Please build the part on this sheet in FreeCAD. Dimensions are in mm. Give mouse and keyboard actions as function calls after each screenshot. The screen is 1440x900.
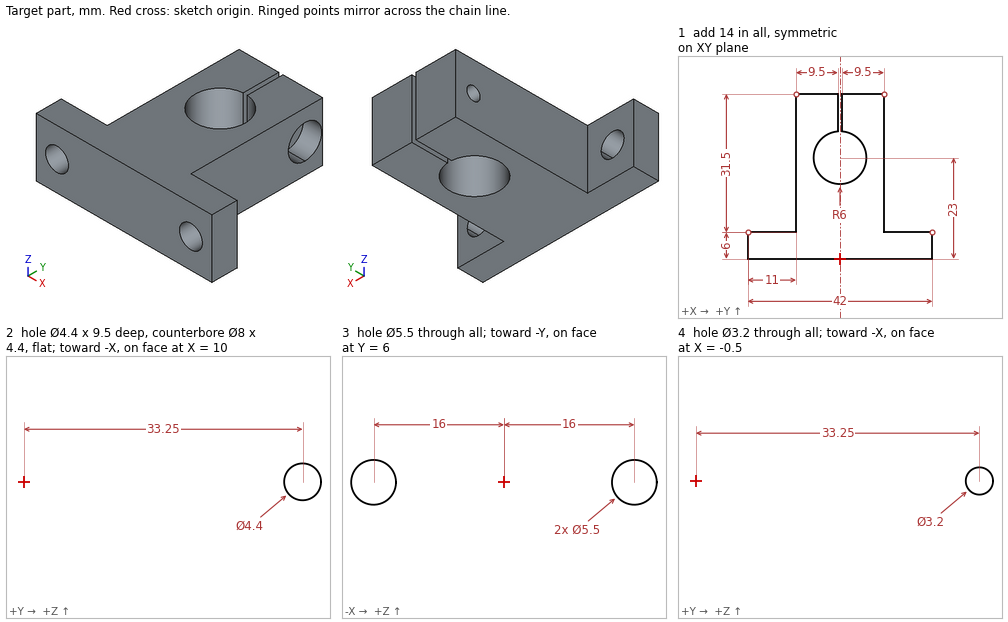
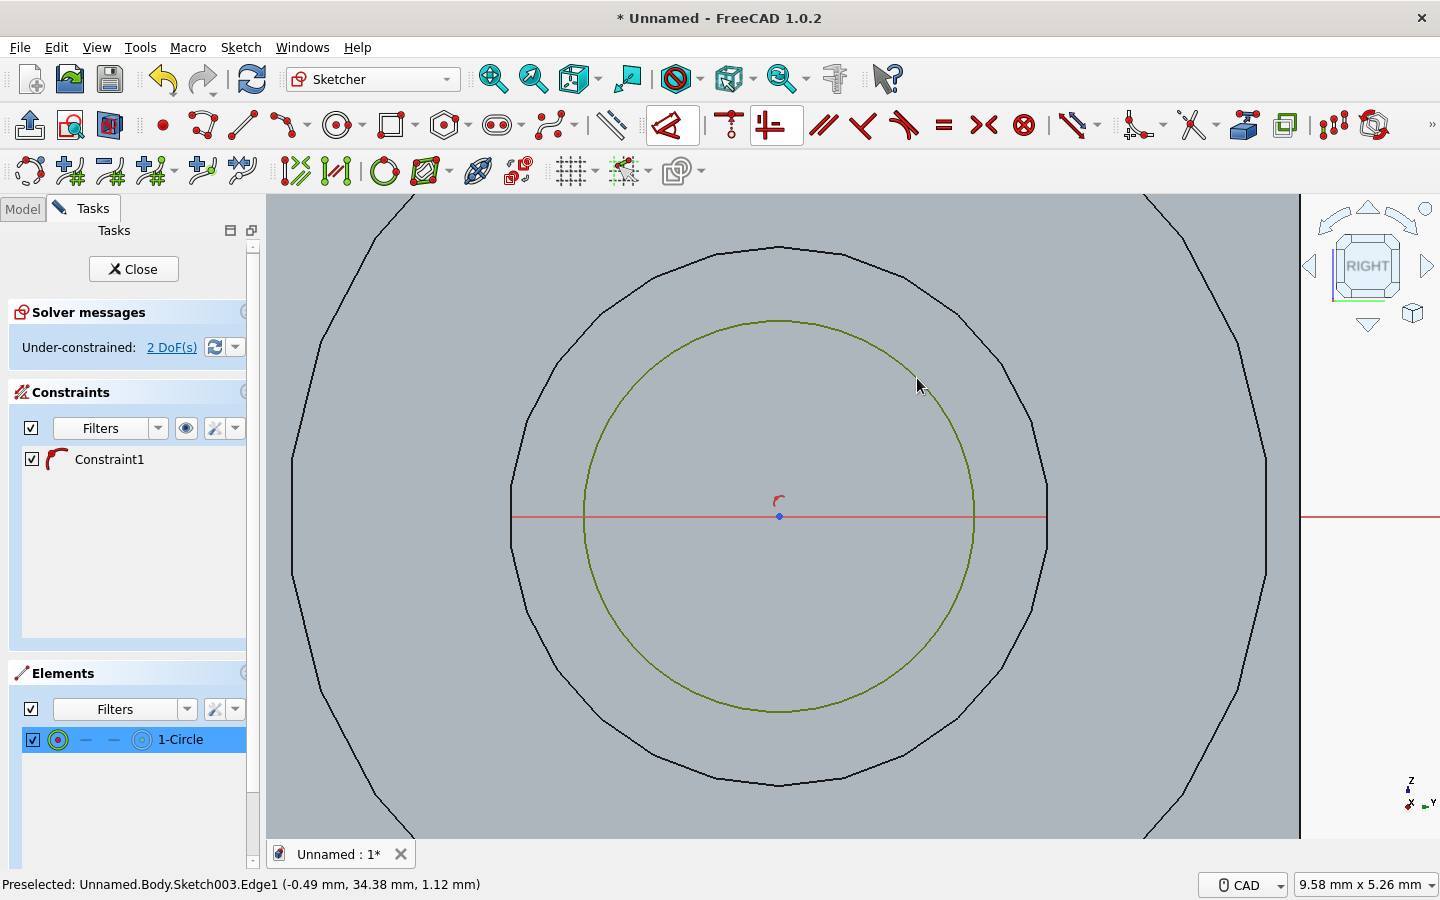
click(694, 126)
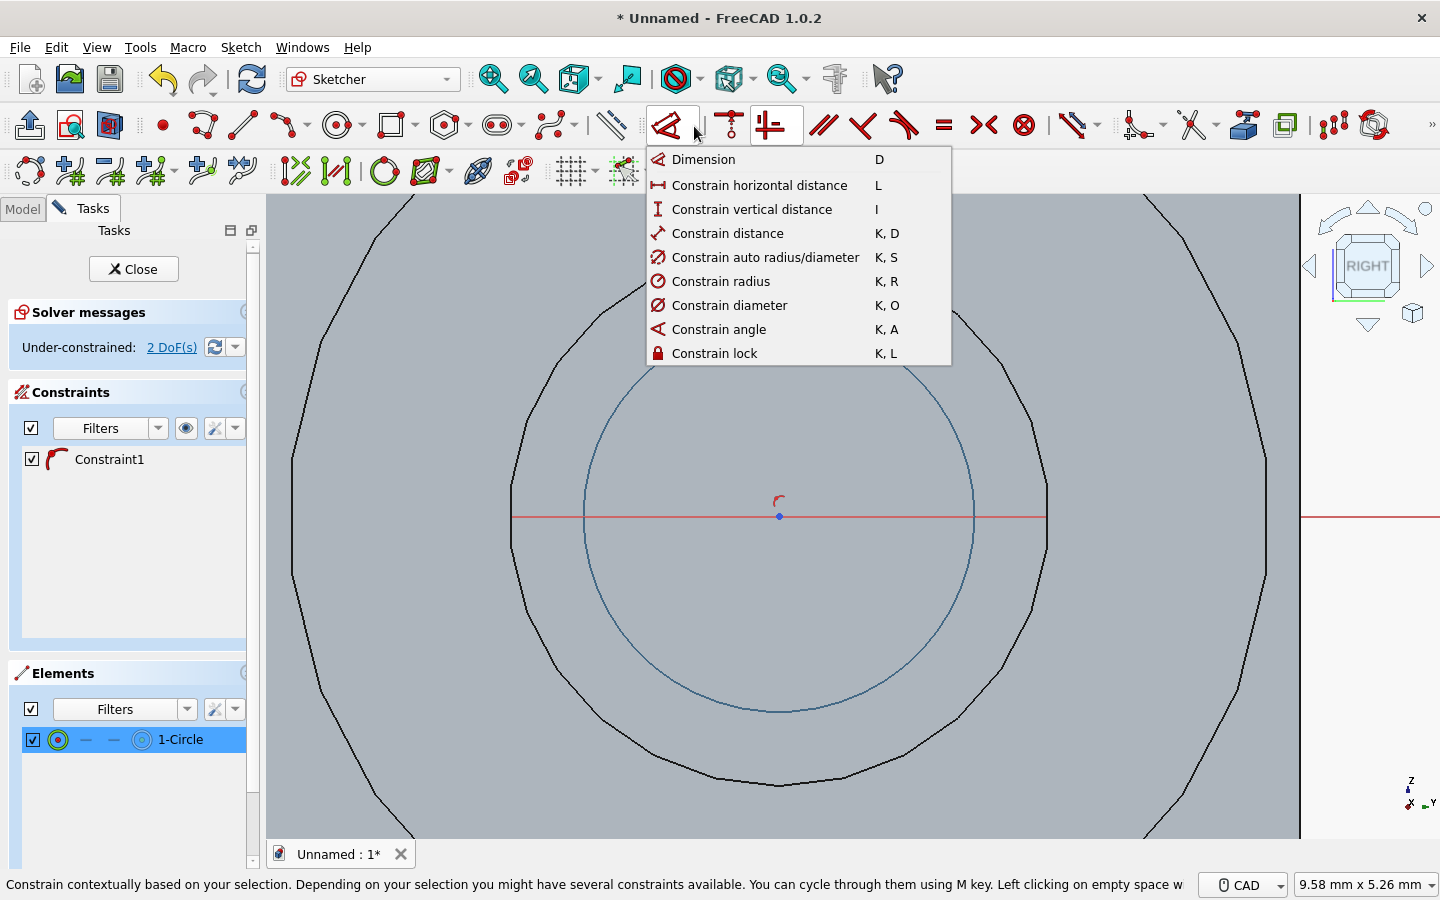
click(799, 305)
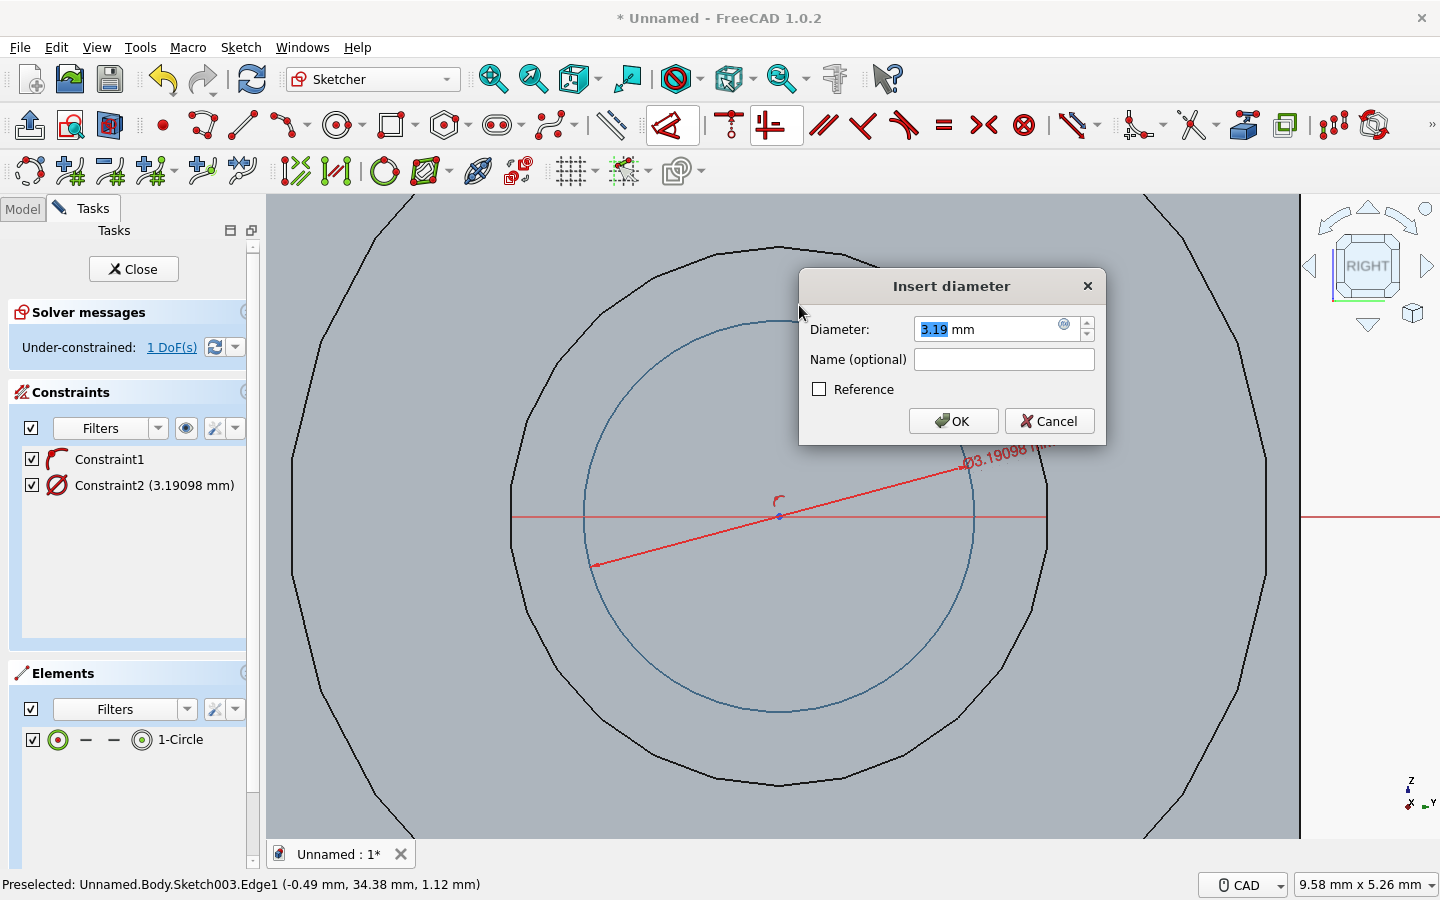
text(3.2)
key(Return)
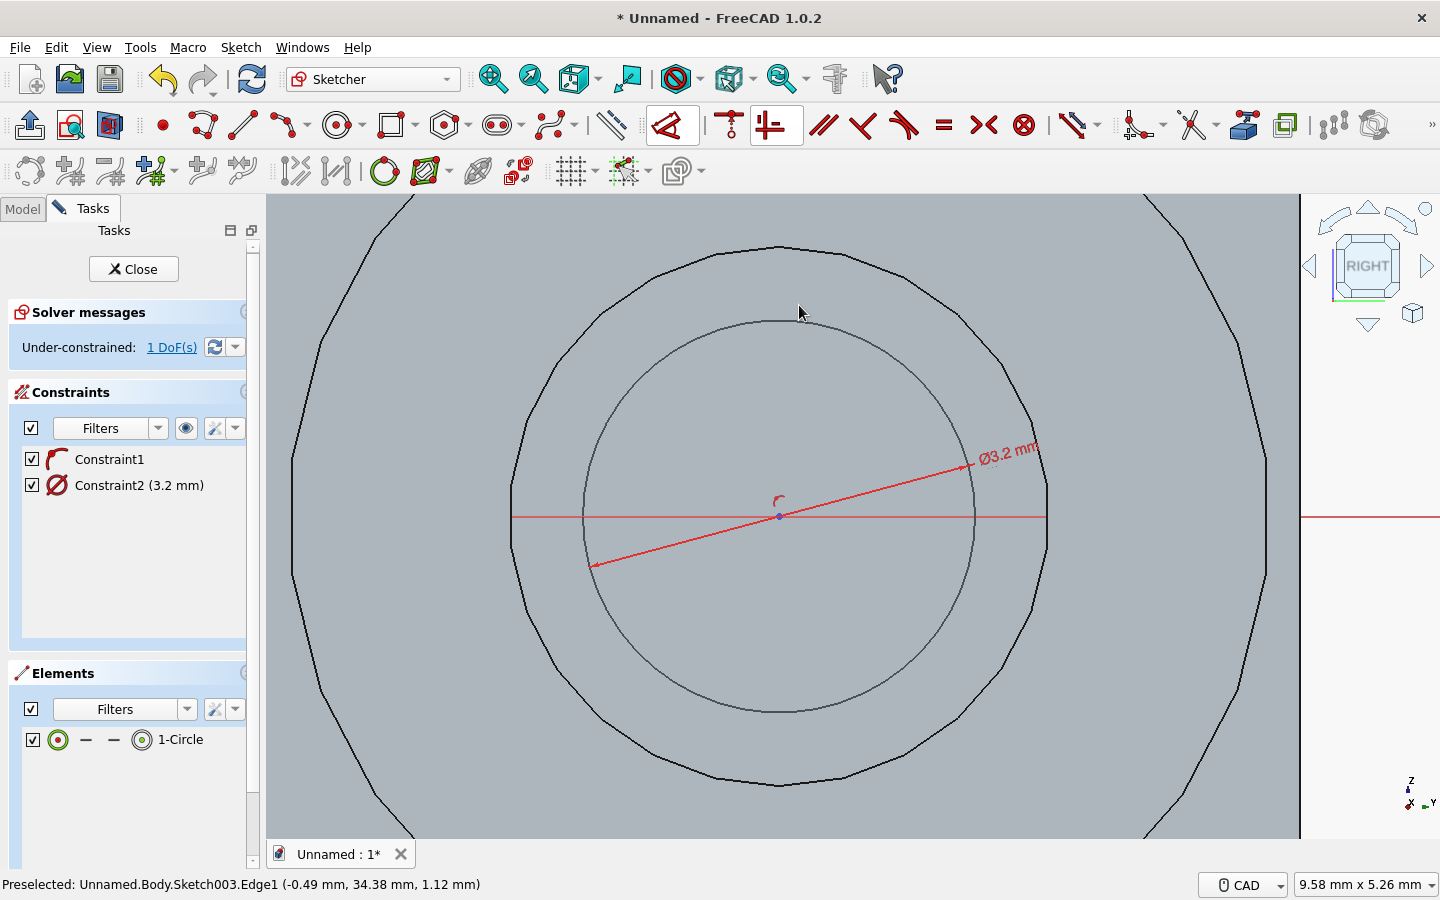
click(779, 516)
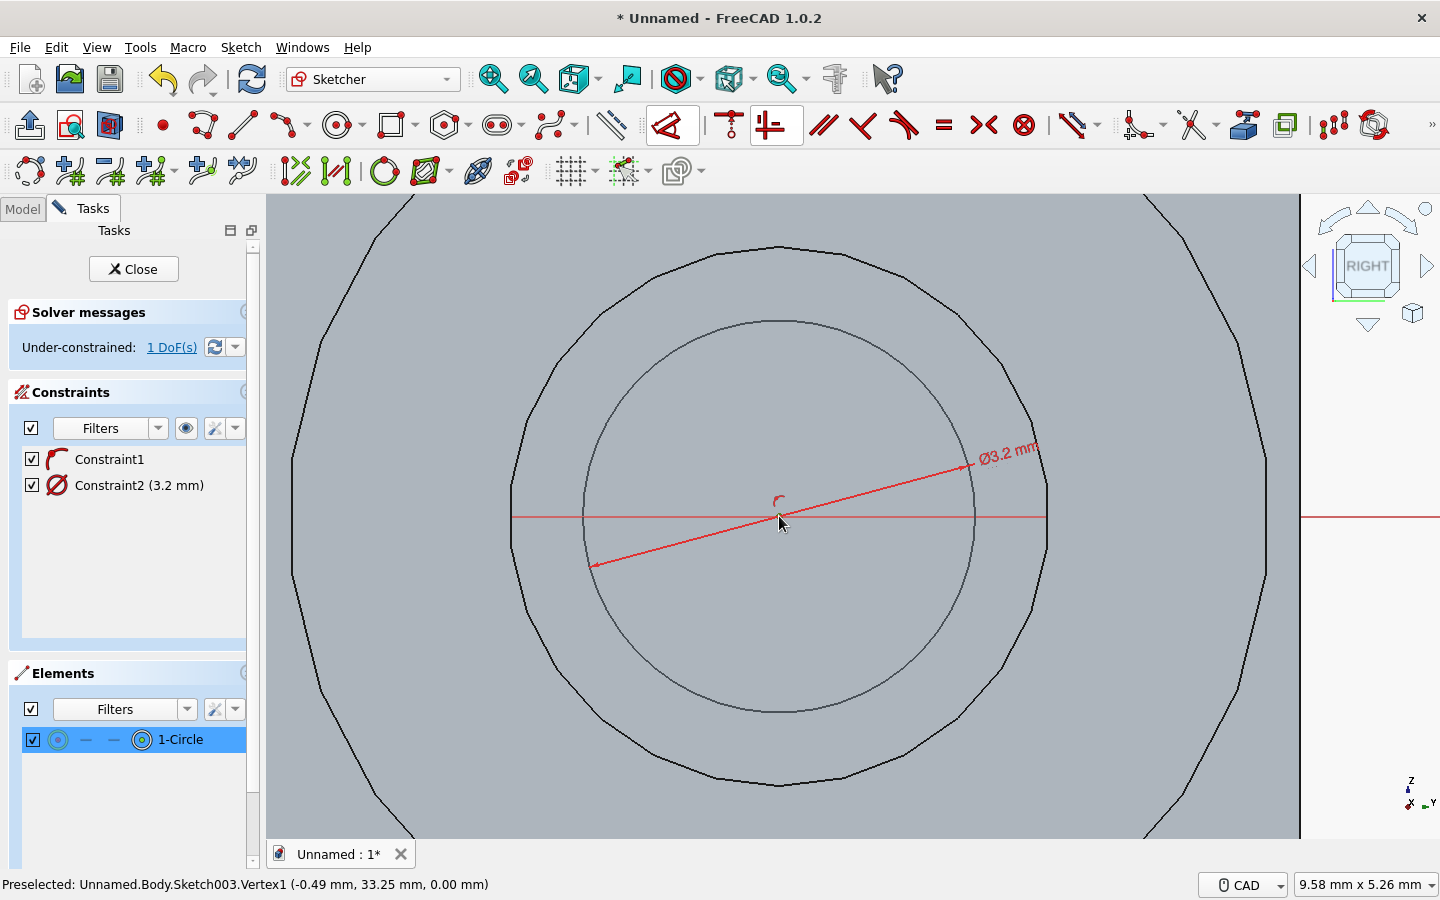
click(694, 126)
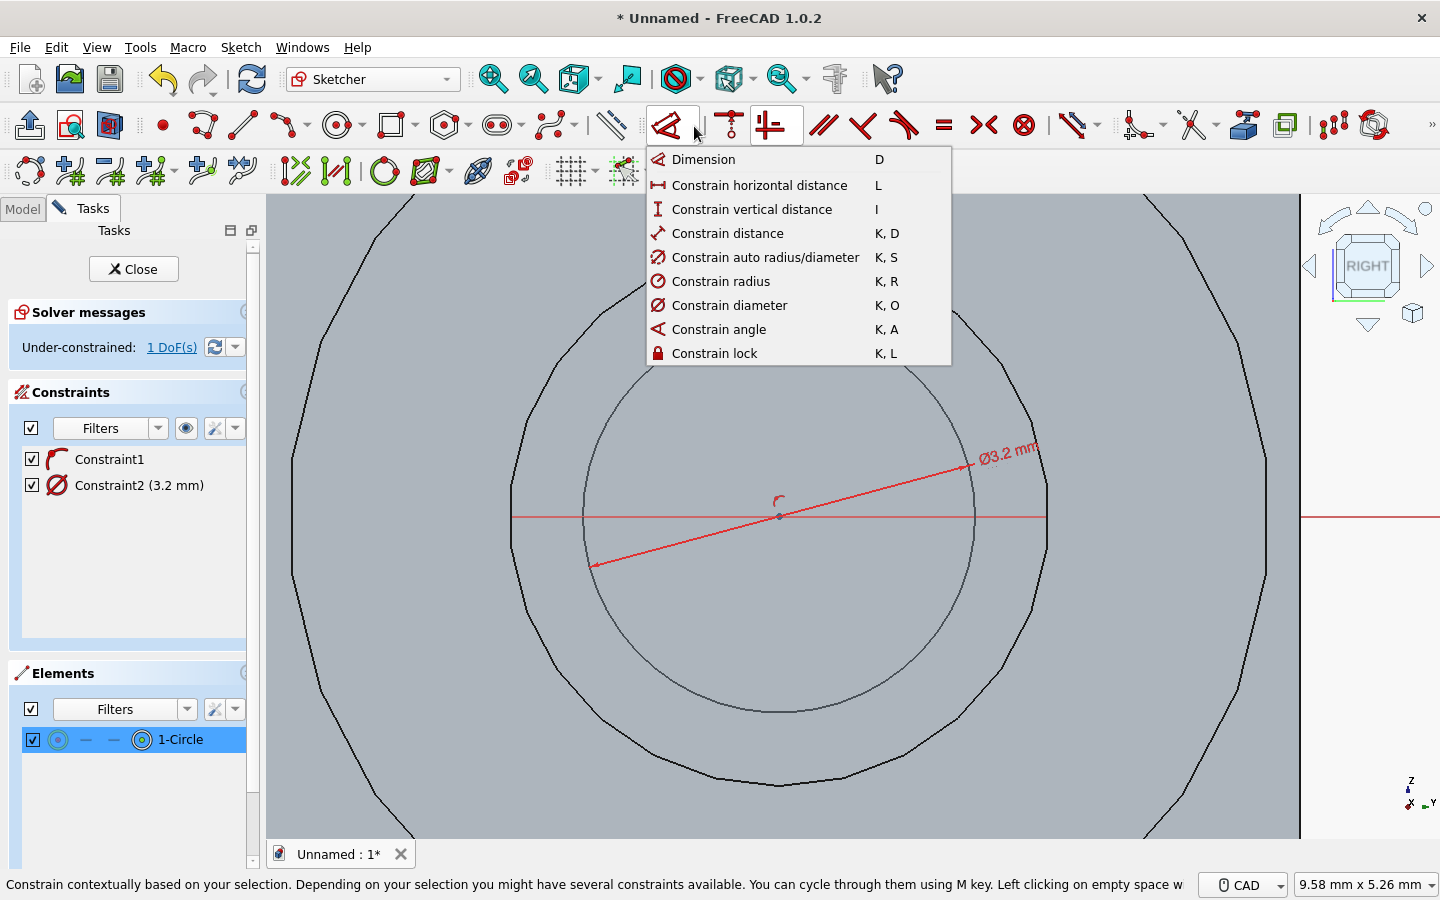
click(799, 185)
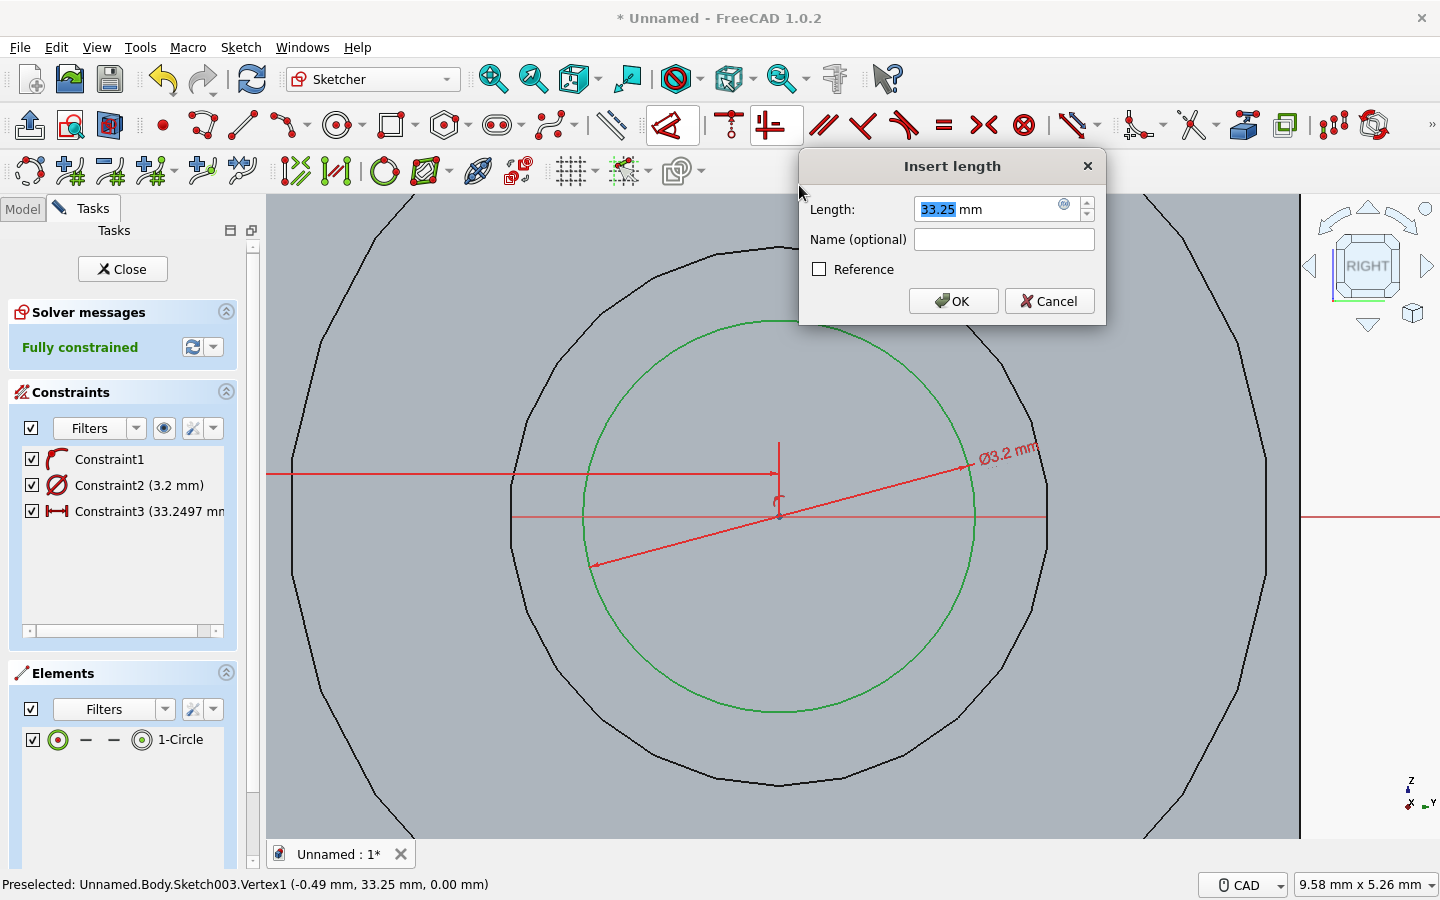
text(33.25)
key(Return)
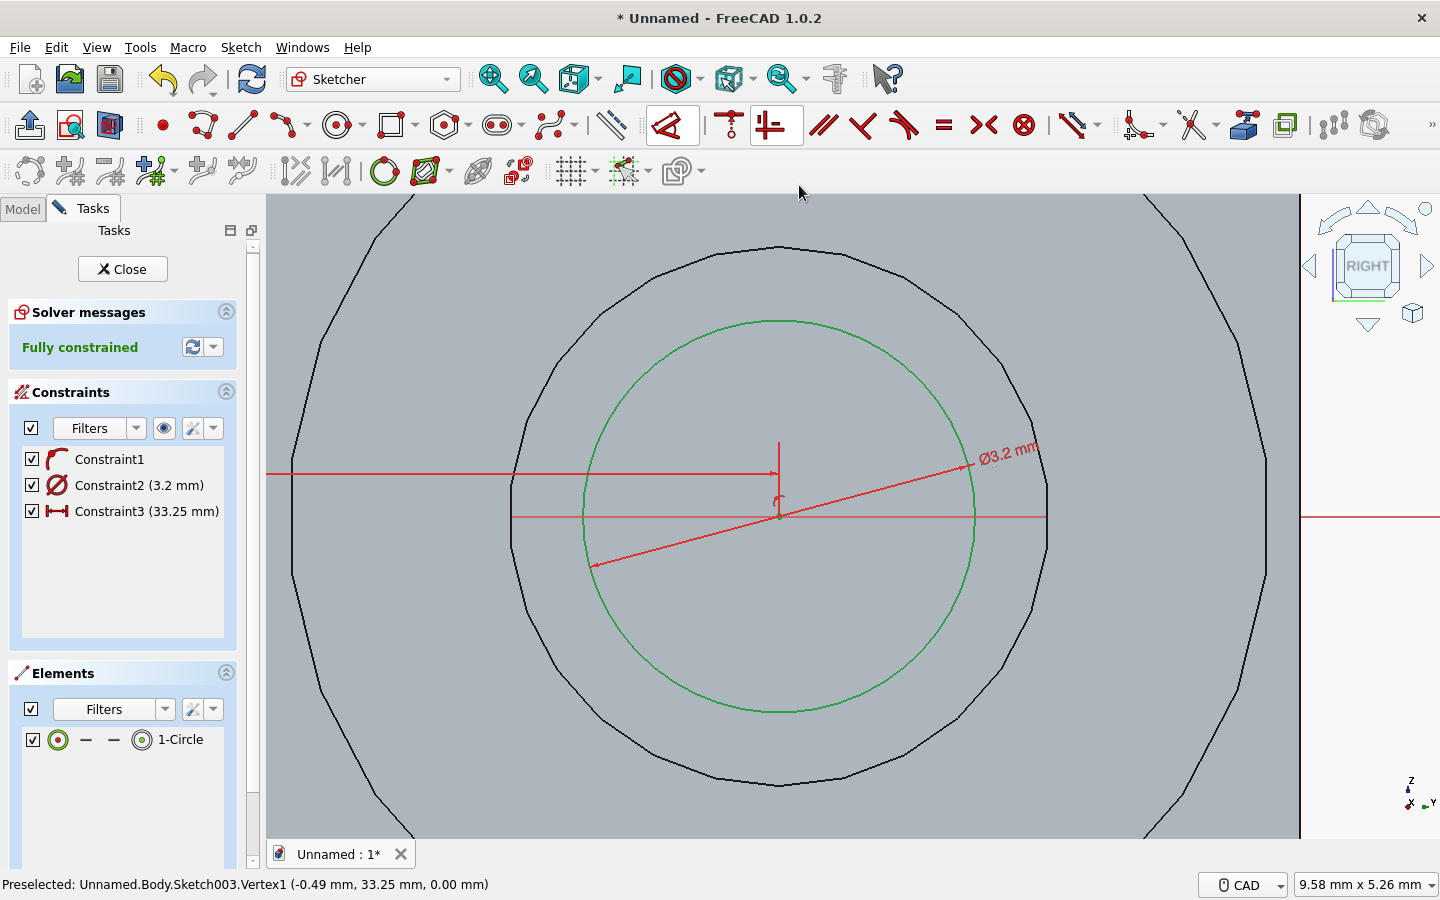
click(123, 269)